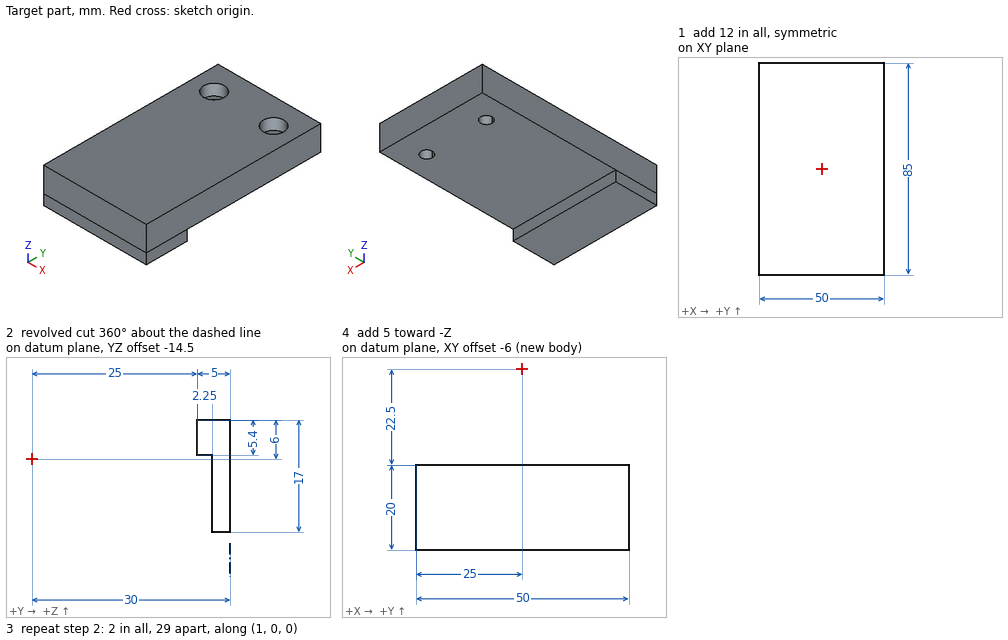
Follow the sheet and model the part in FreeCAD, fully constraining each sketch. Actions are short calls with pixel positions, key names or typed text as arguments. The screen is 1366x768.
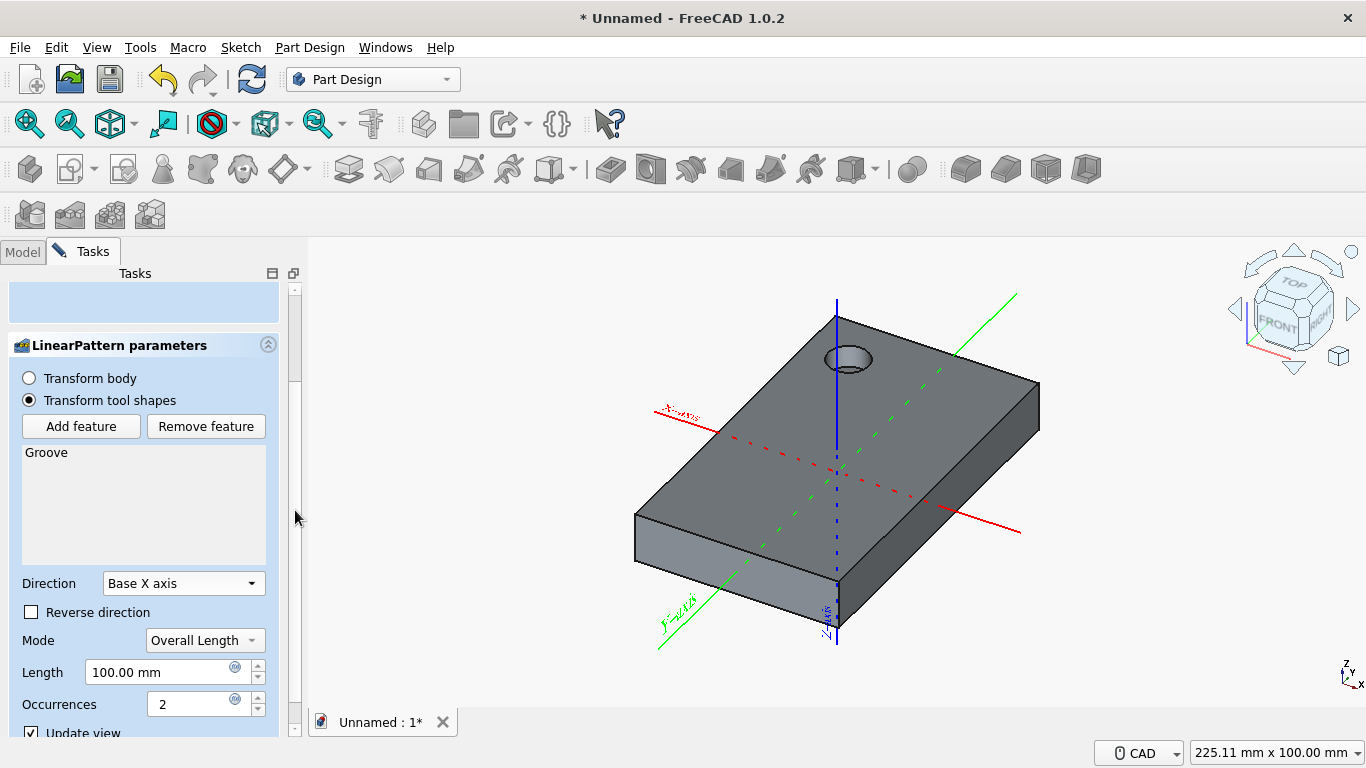
click(206, 640)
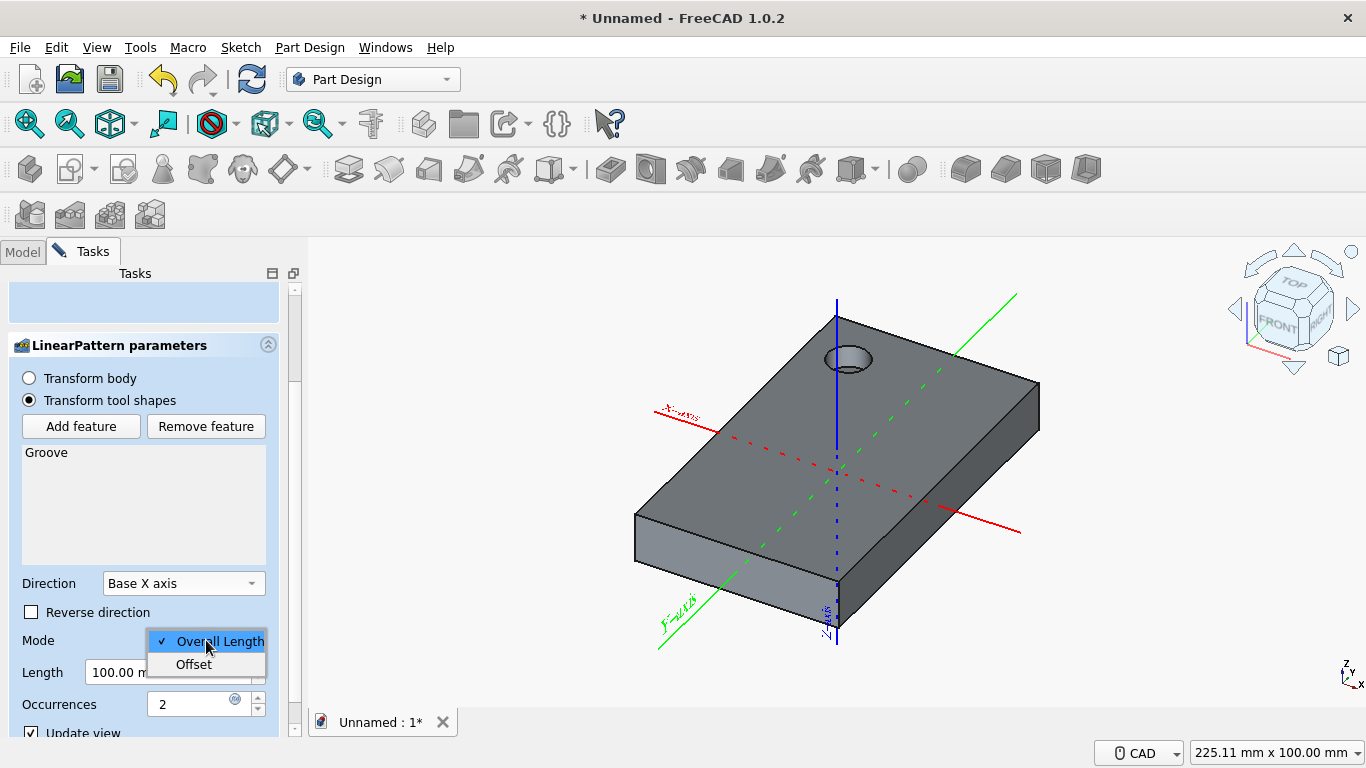
click(206, 664)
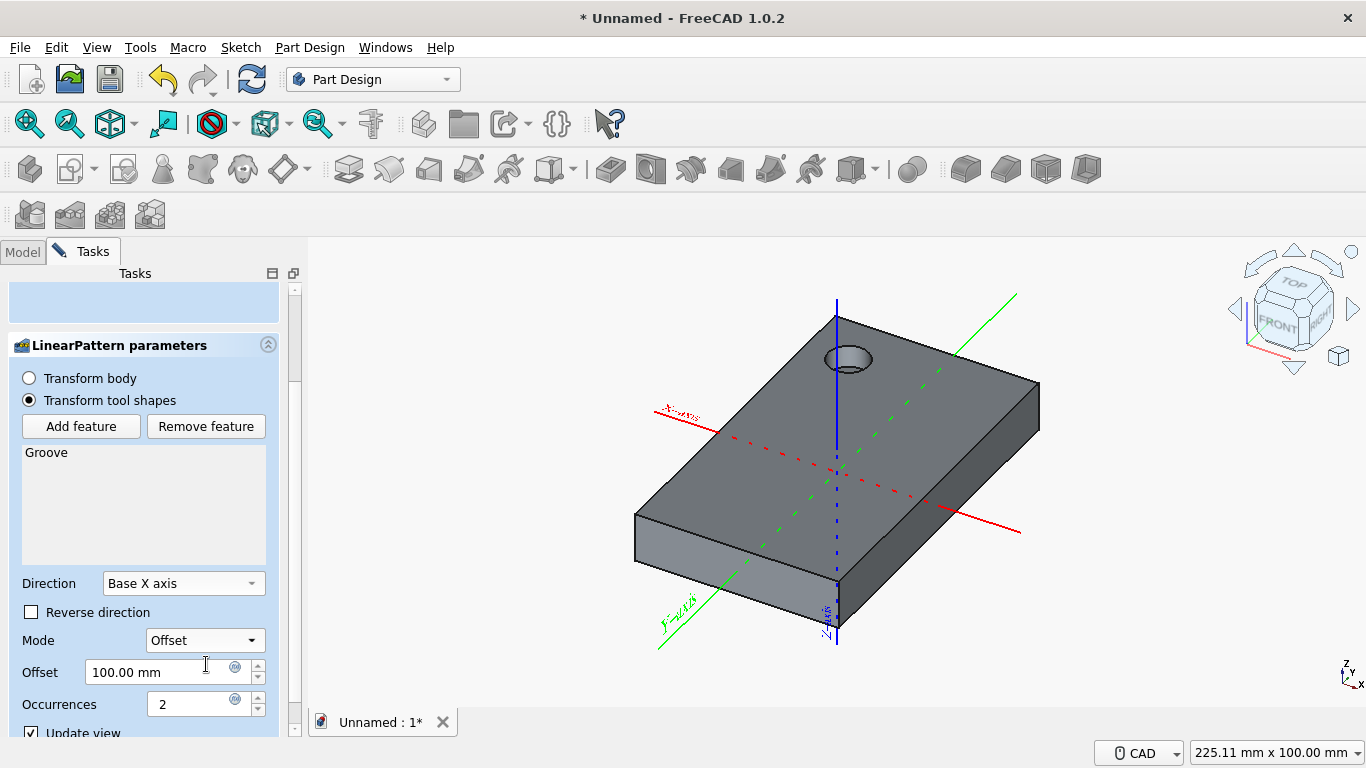
triple_click(168, 672)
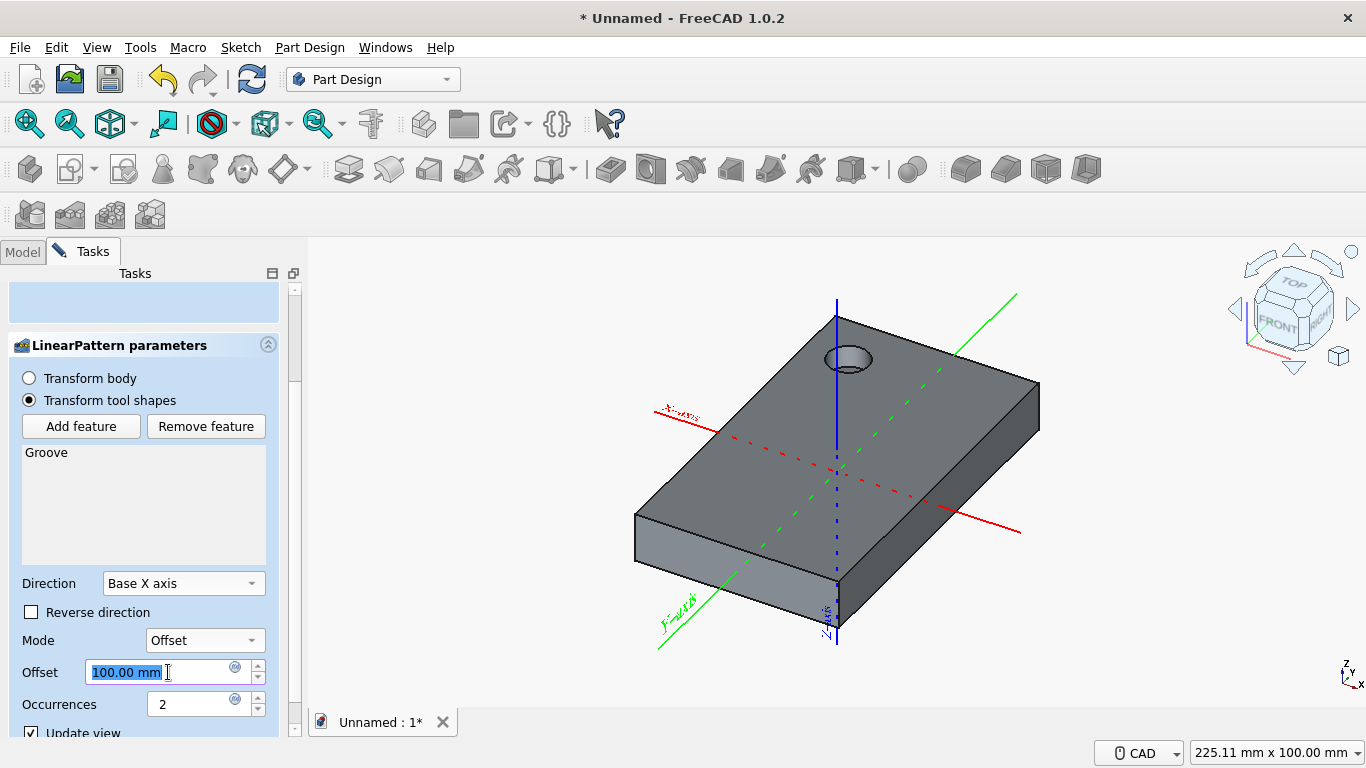
text(29)
key(Tab)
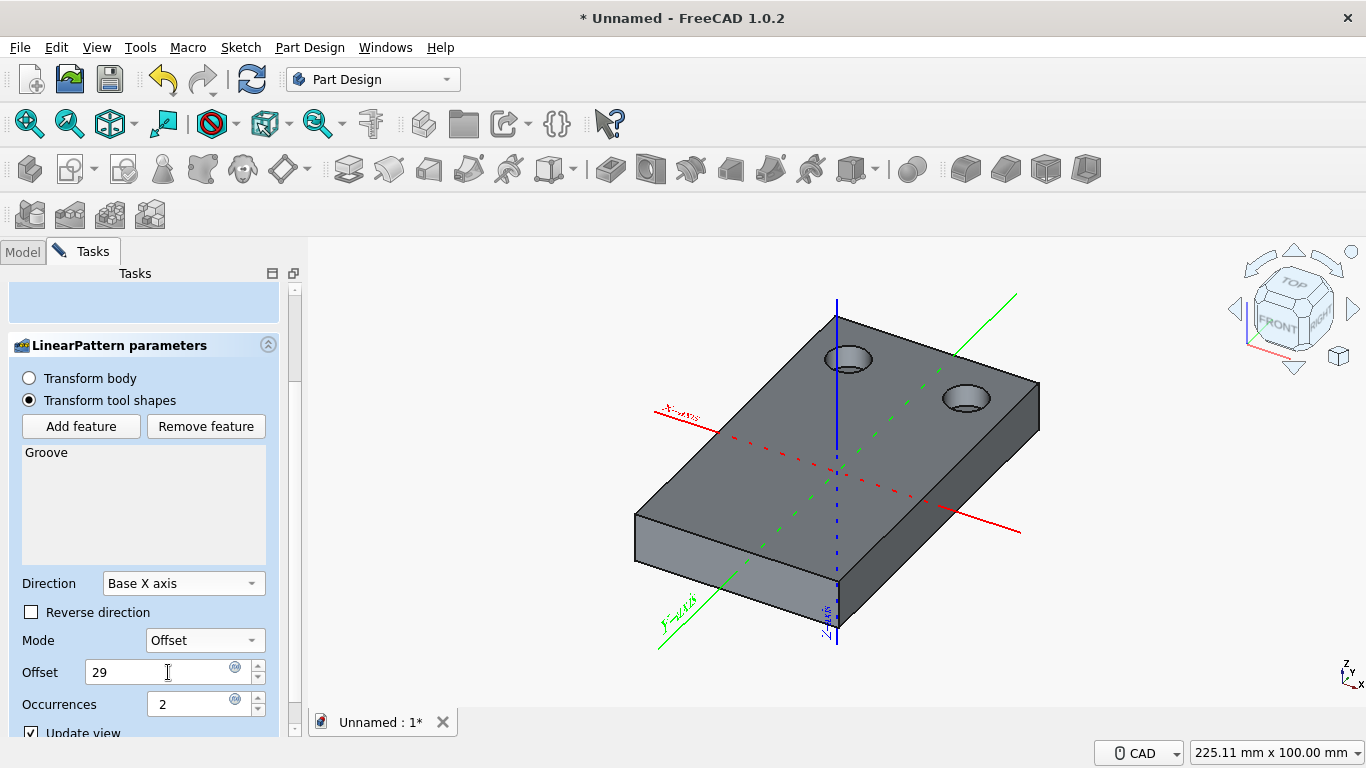
triple_click(198, 704)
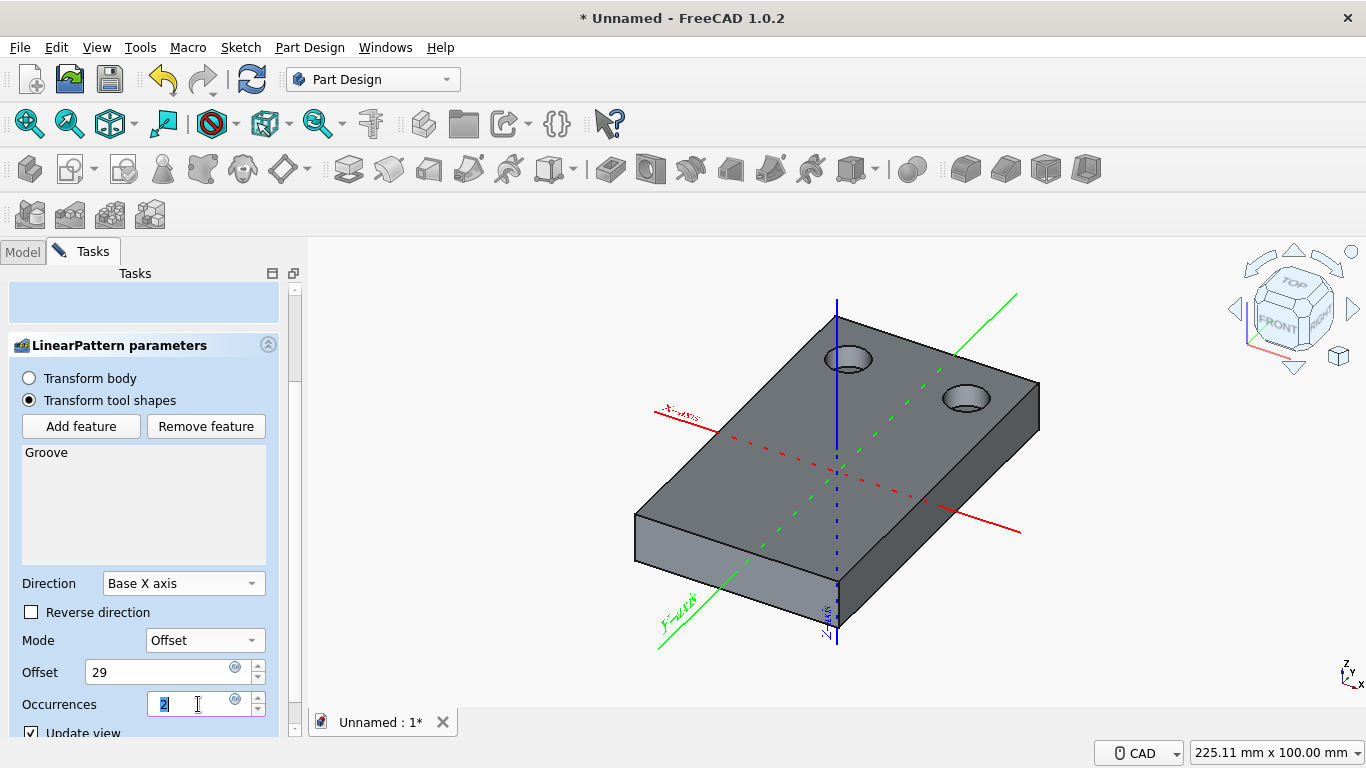
text(2)
key(Tab)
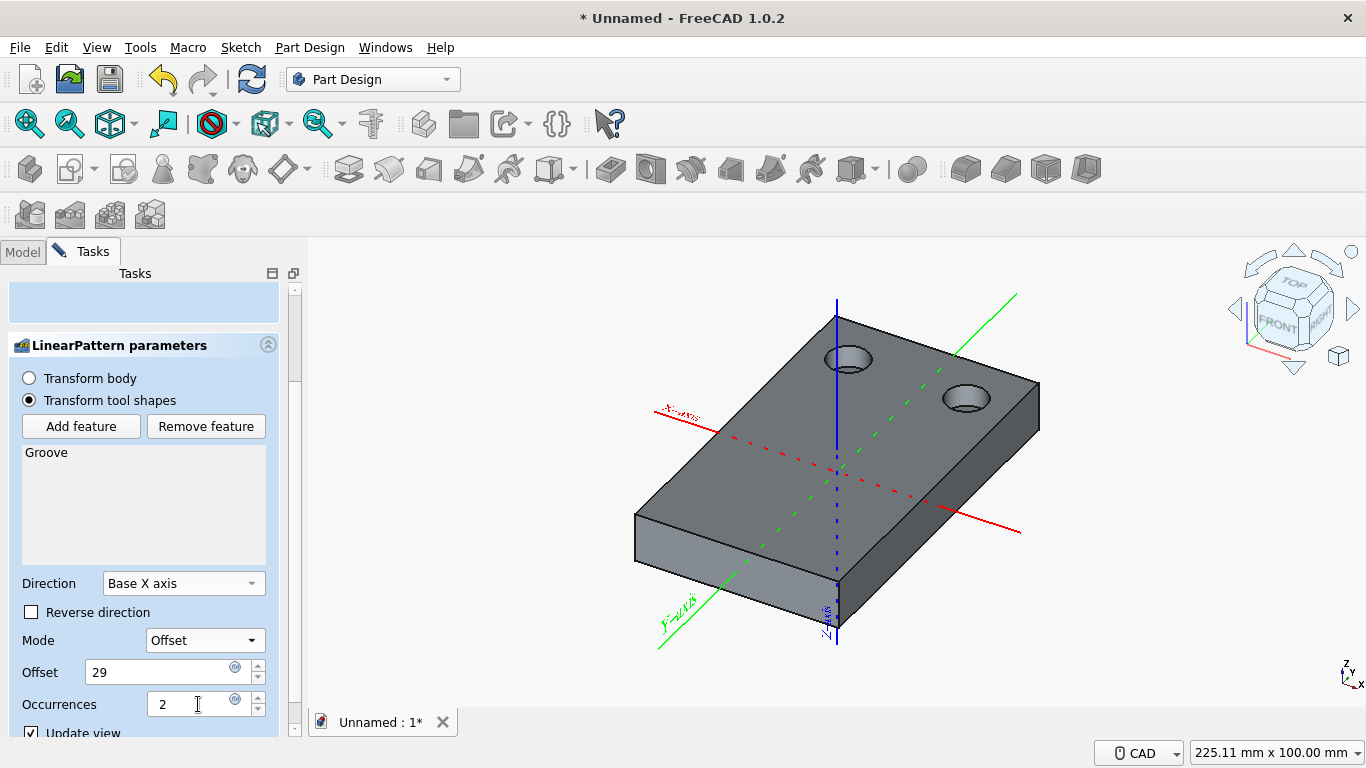
scroll(295, 510, up, 3)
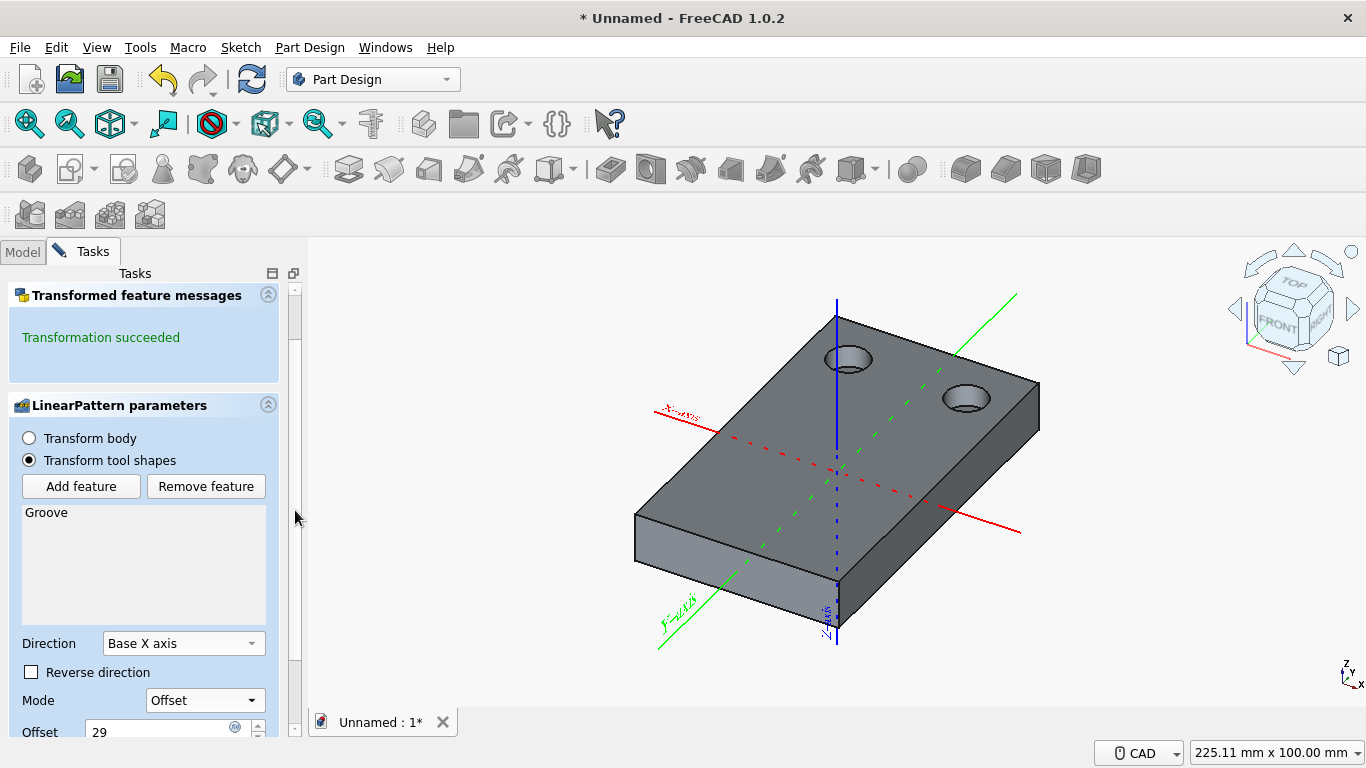
click(96, 312)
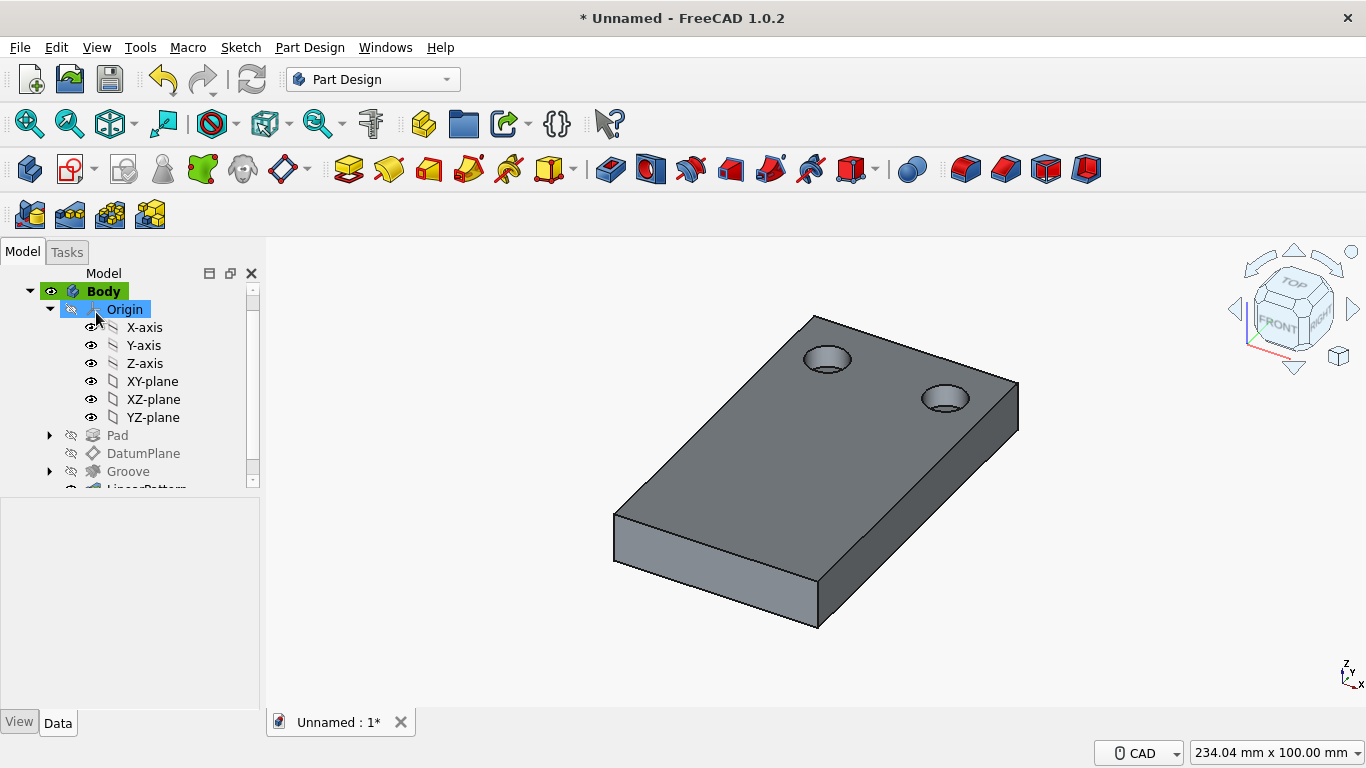
click(30, 170)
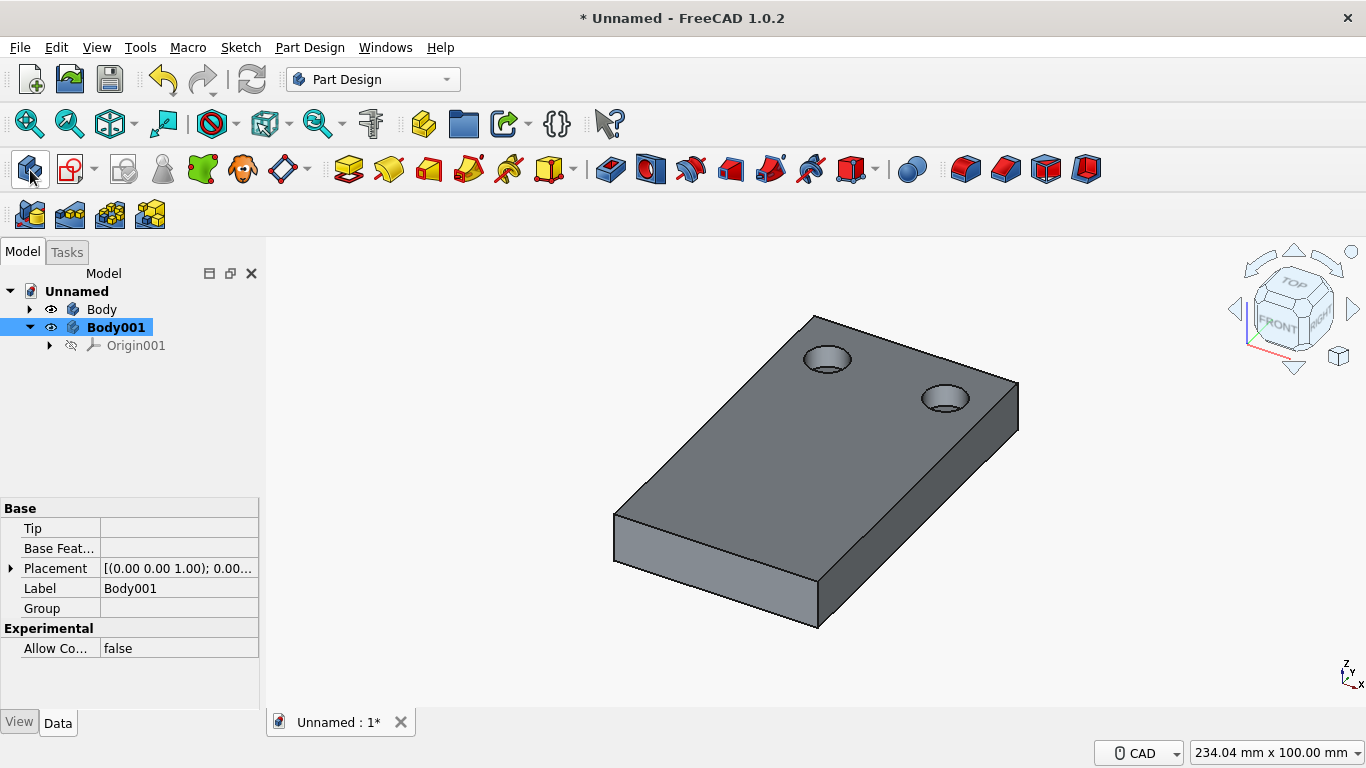
click(50, 345)